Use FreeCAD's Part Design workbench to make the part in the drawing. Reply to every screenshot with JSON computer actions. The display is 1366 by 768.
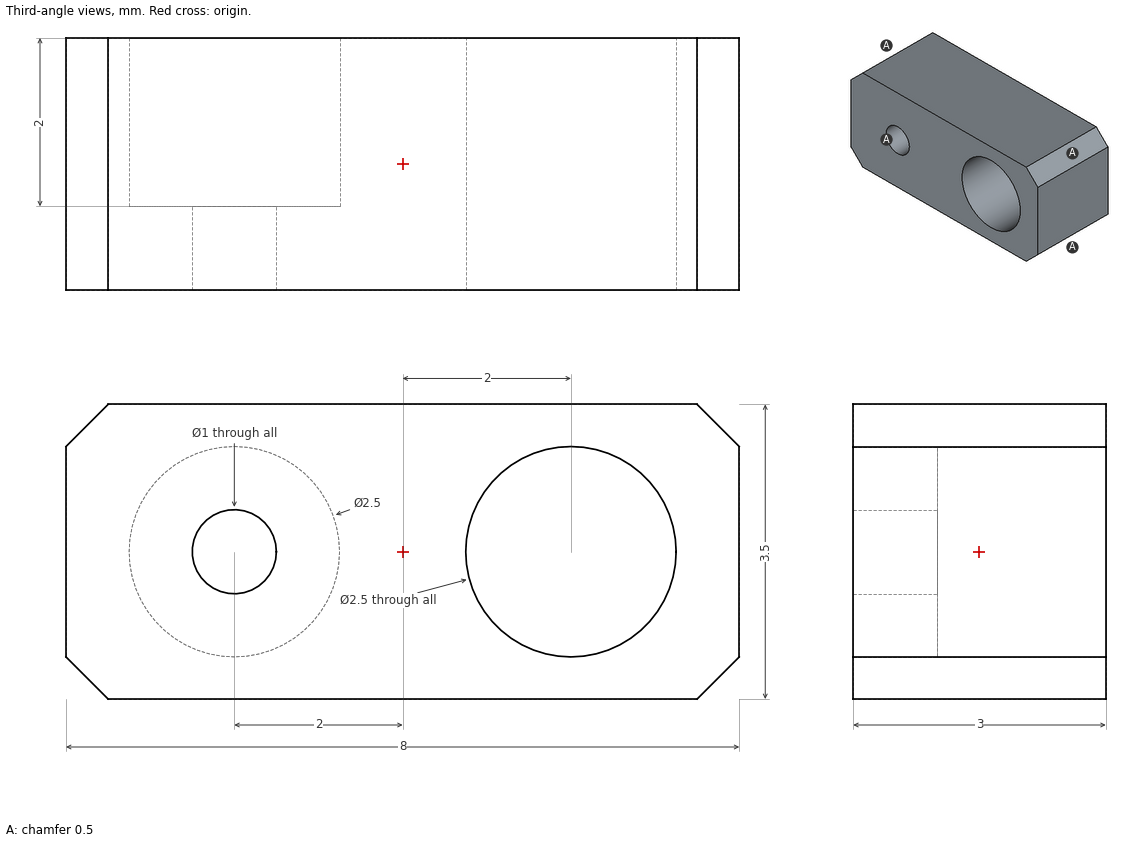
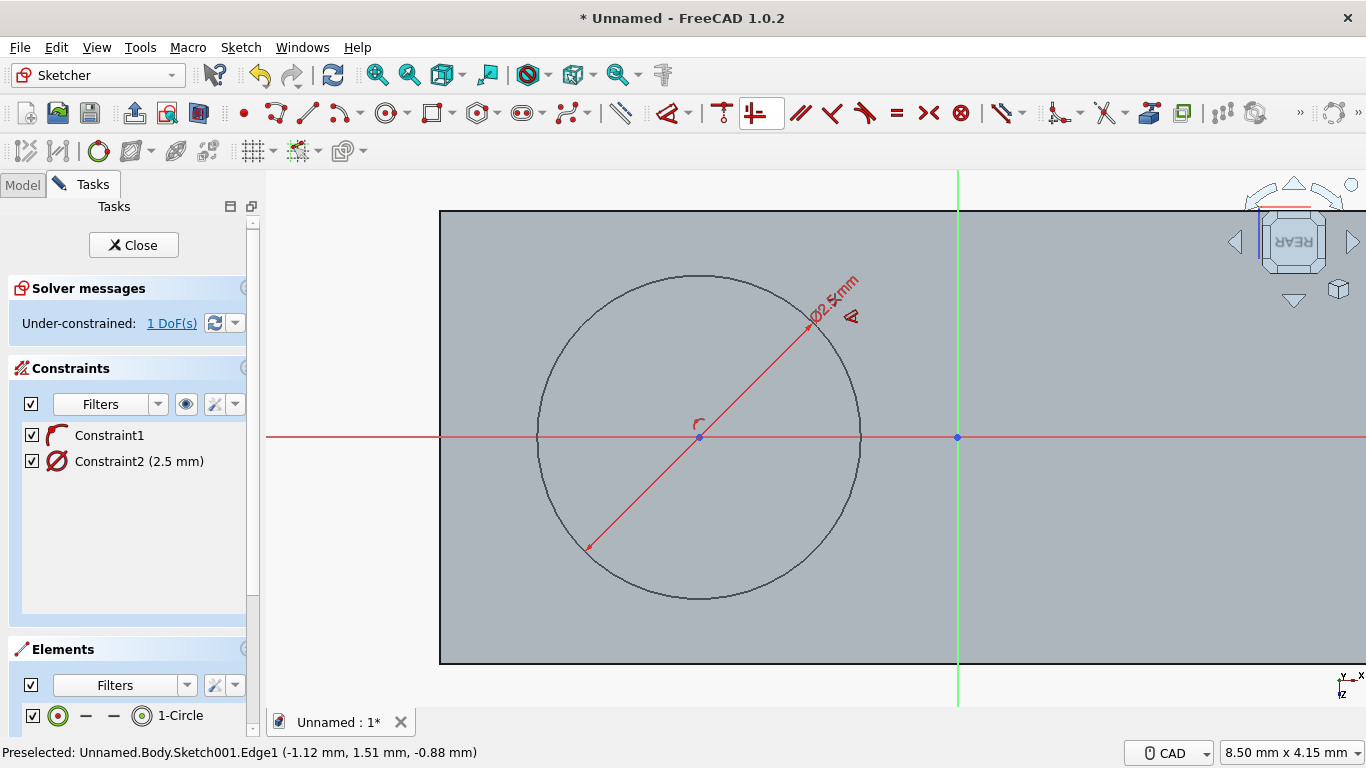
{"action": "left_click", "coordinate": [699, 437]}
{"action": "left_click", "coordinate": [828, 471]}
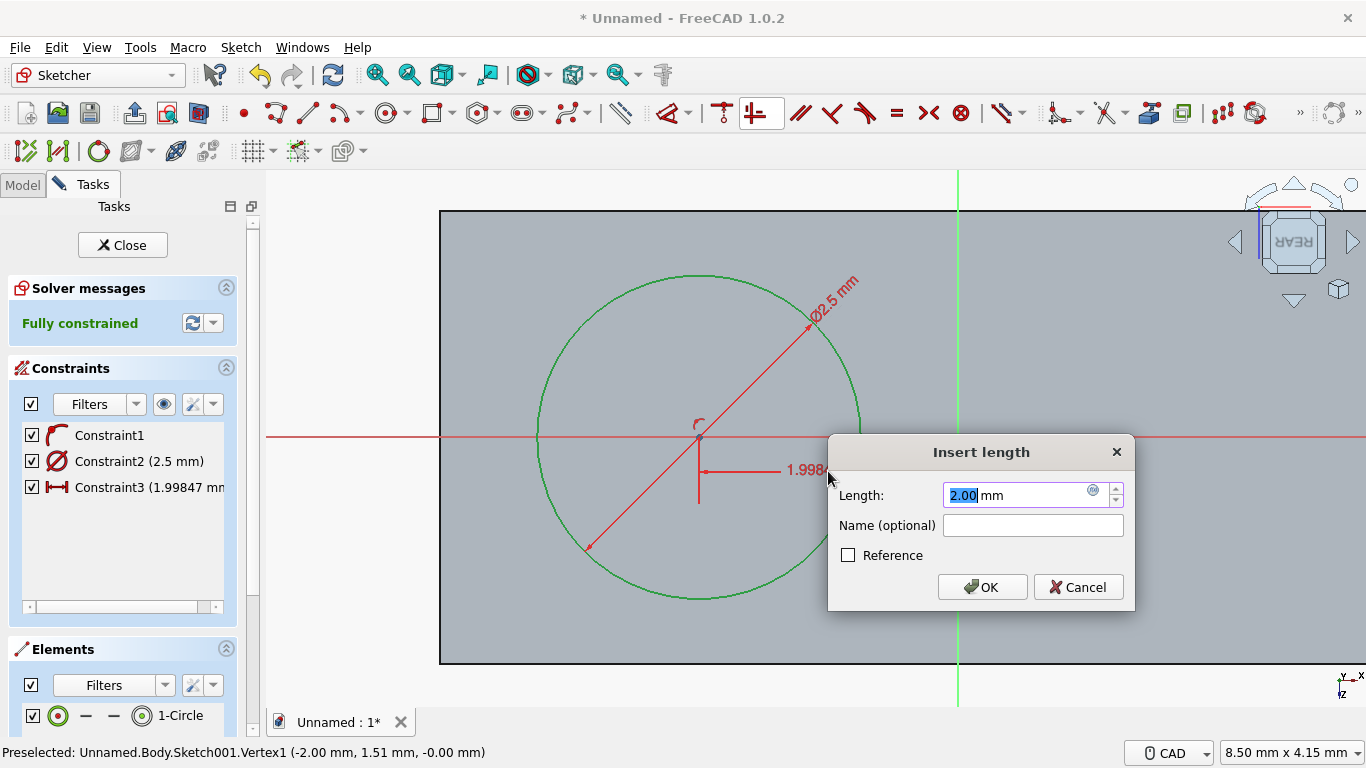
{"action": "type", "text": "2"}
{"action": "key", "text": "Return"}
{"action": "key", "text": "Escape"}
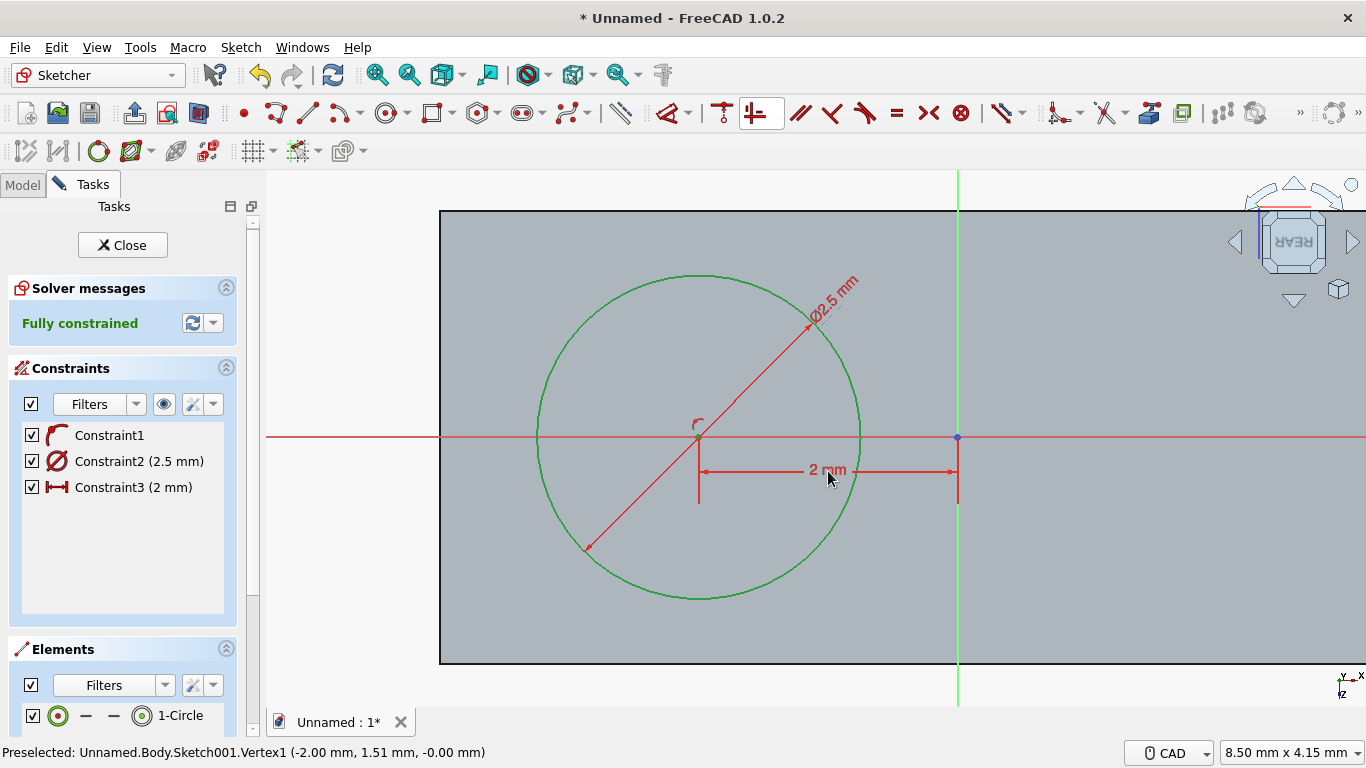
{"action": "left_click", "coordinate": [123, 245]}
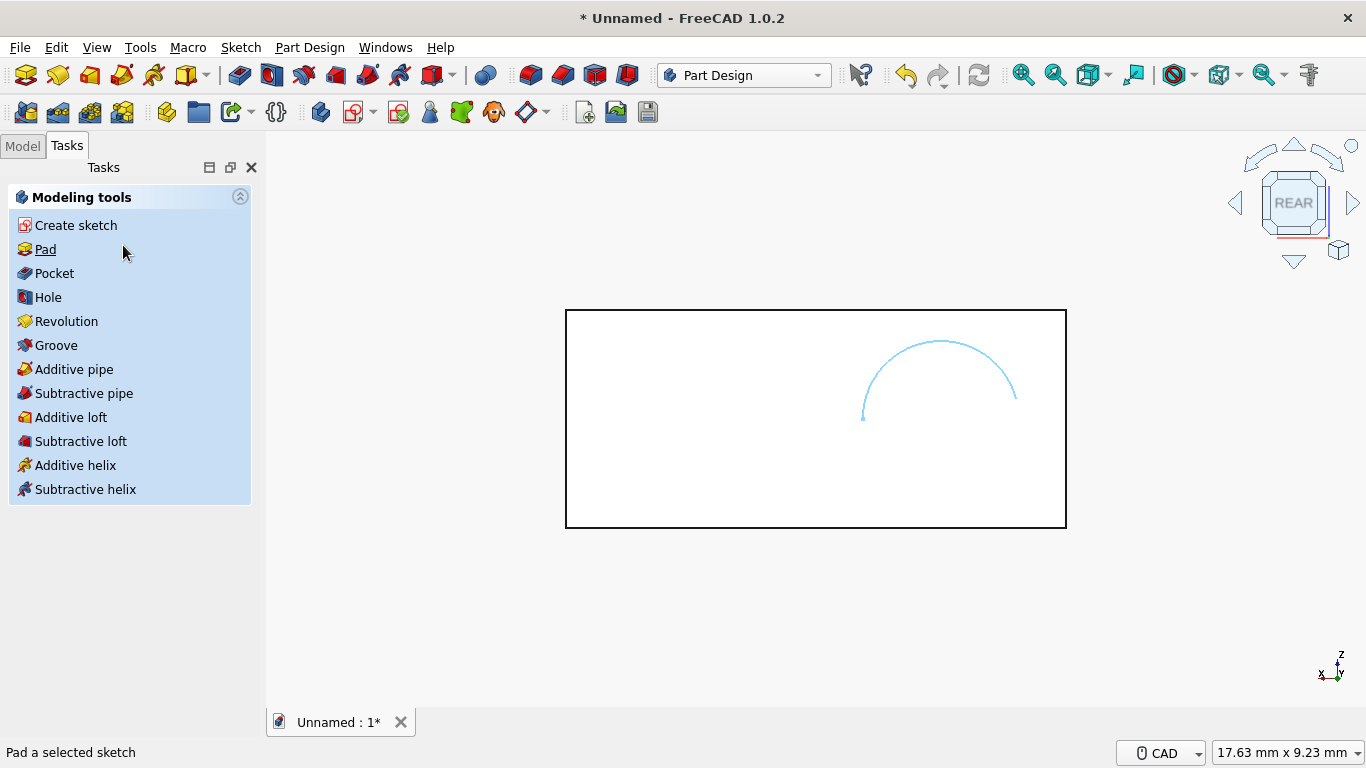
{"action": "left_click", "coordinate": [240, 76]}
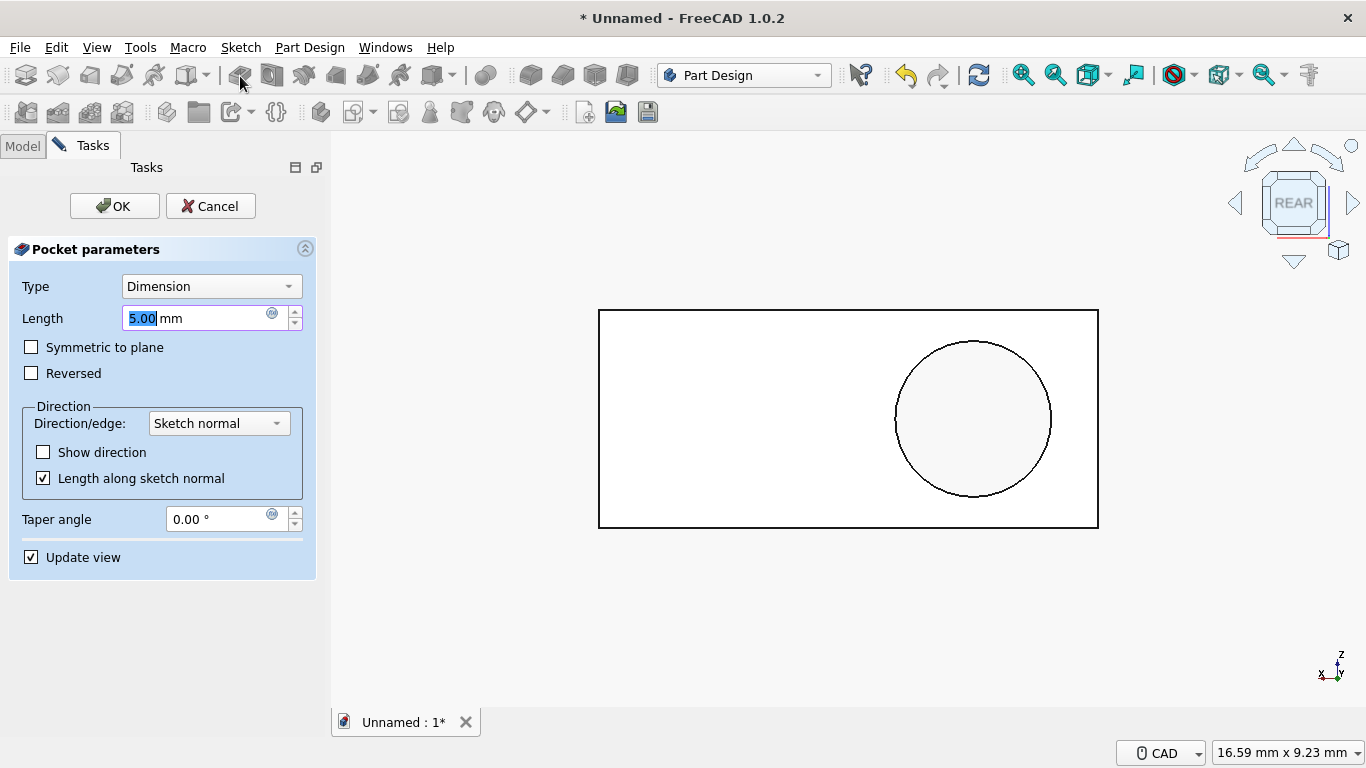
{"action": "type", "text": "2"}
{"action": "key", "text": "Tab"}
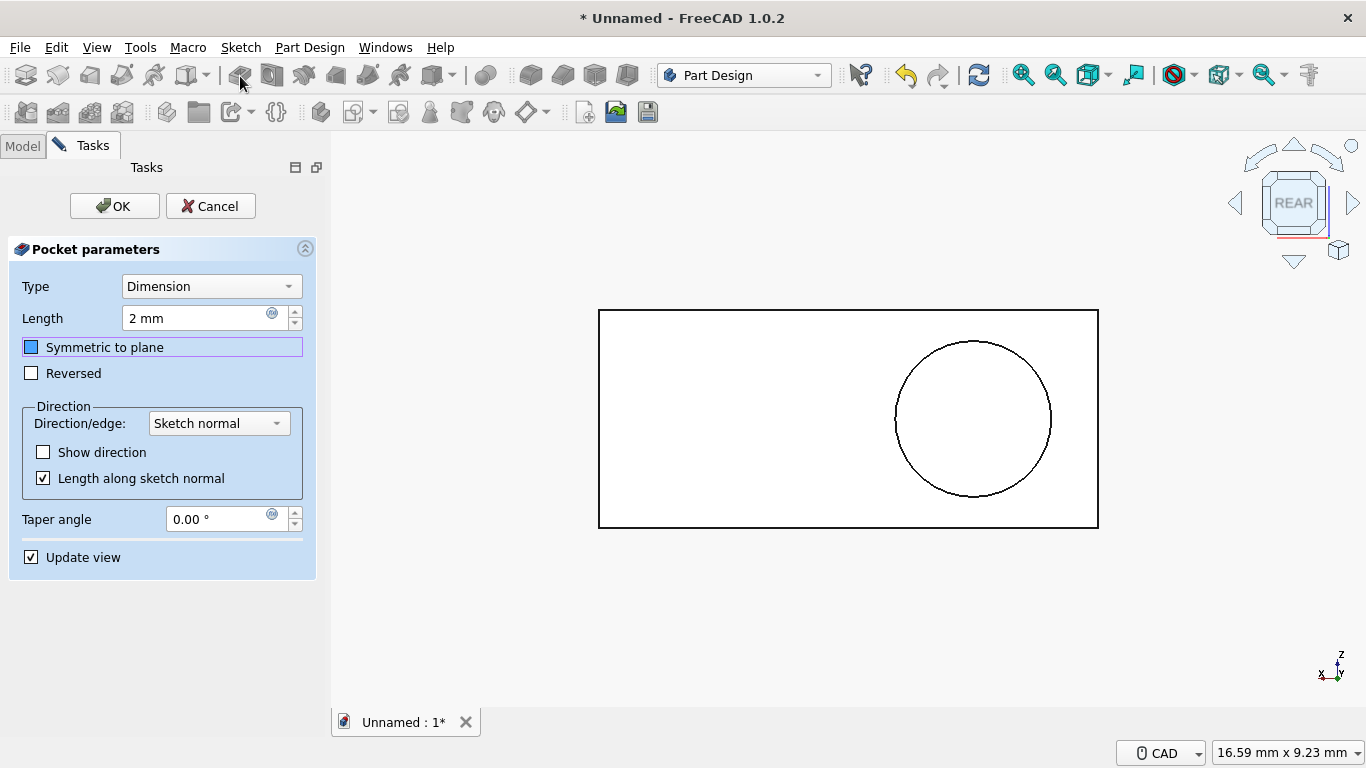
{"action": "left_click", "coordinate": [115, 206]}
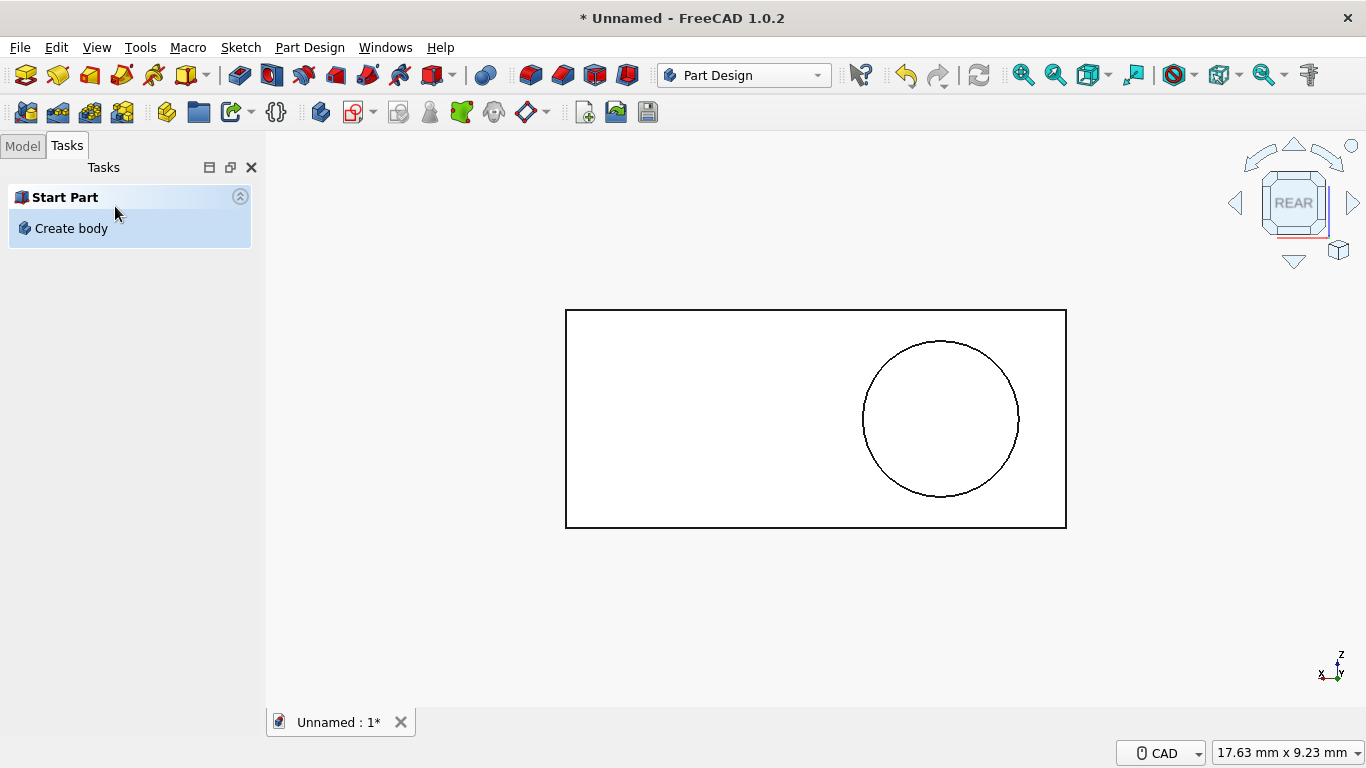
{"action": "key", "text": "0"}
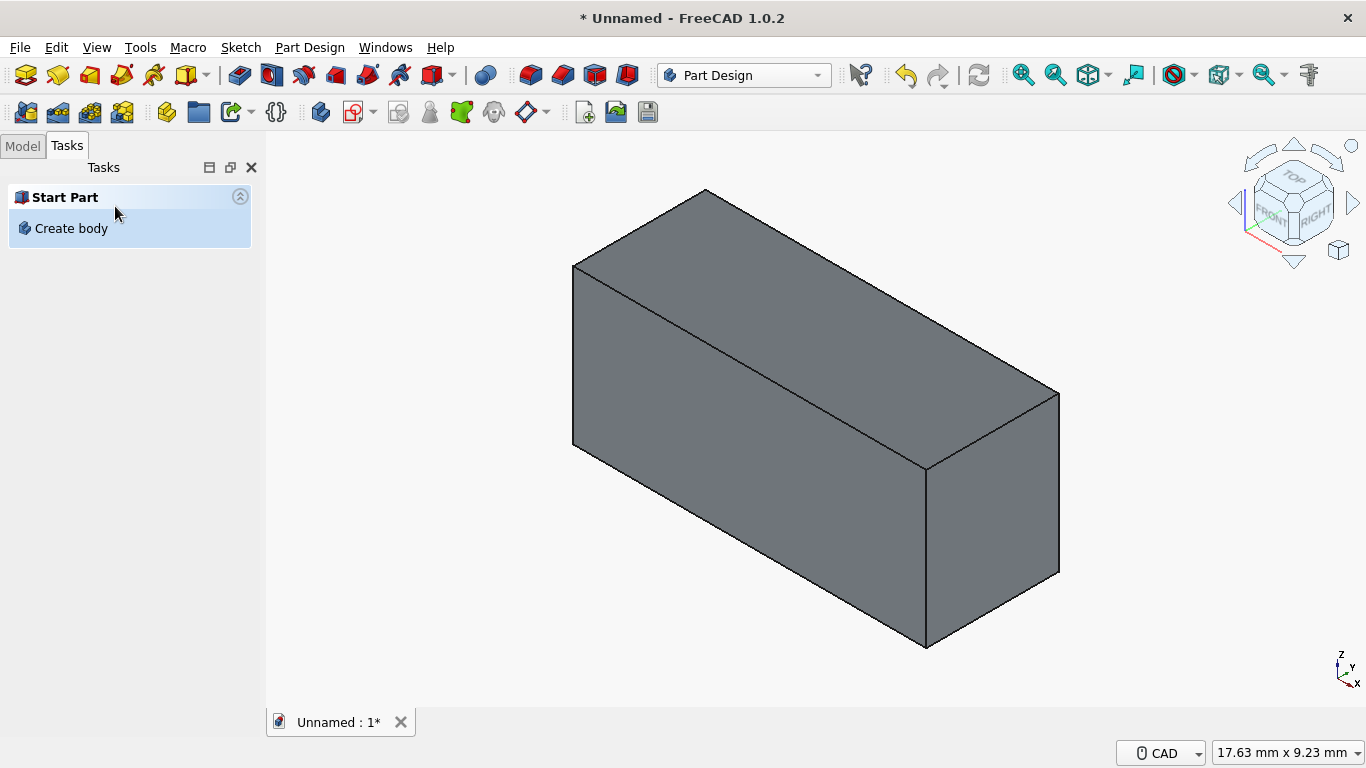
{"action": "left_click", "coordinate": [992, 431]}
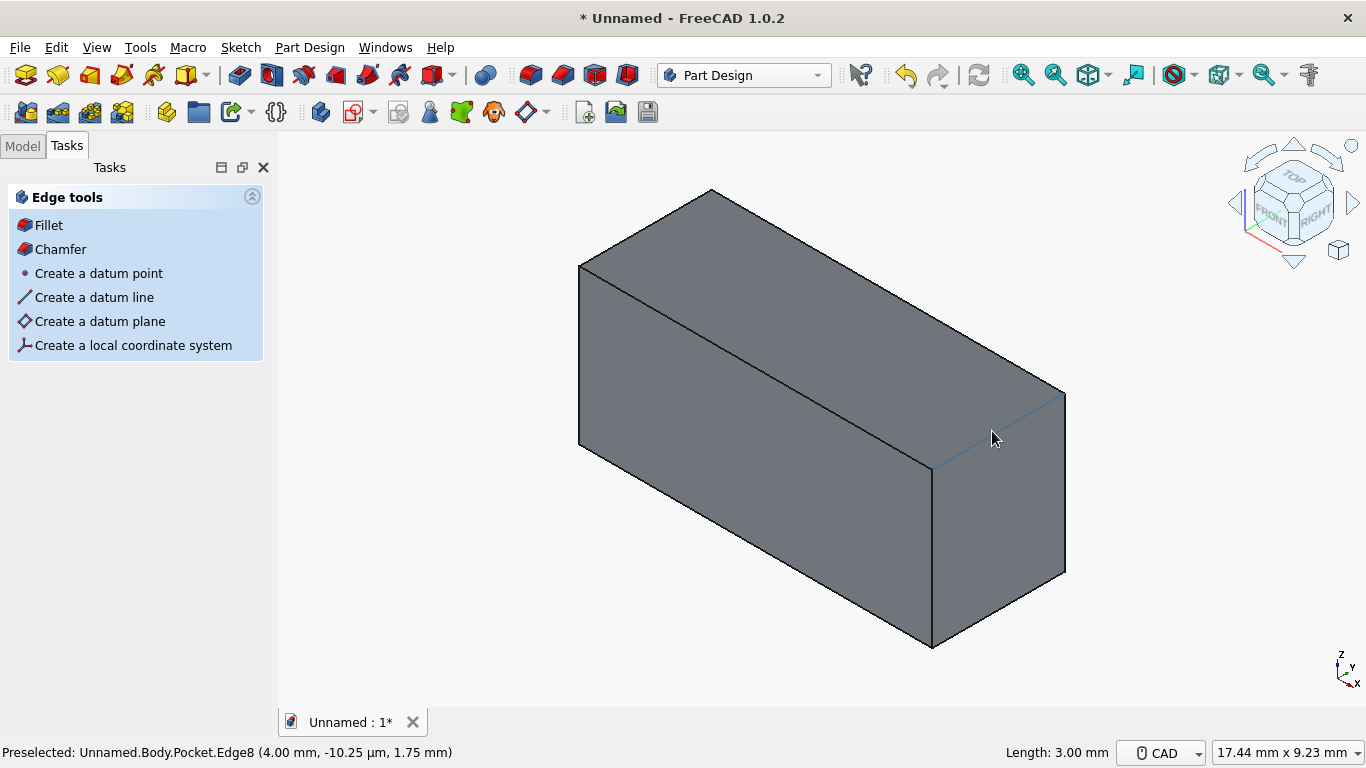
{"action": "key", "text": "2"}